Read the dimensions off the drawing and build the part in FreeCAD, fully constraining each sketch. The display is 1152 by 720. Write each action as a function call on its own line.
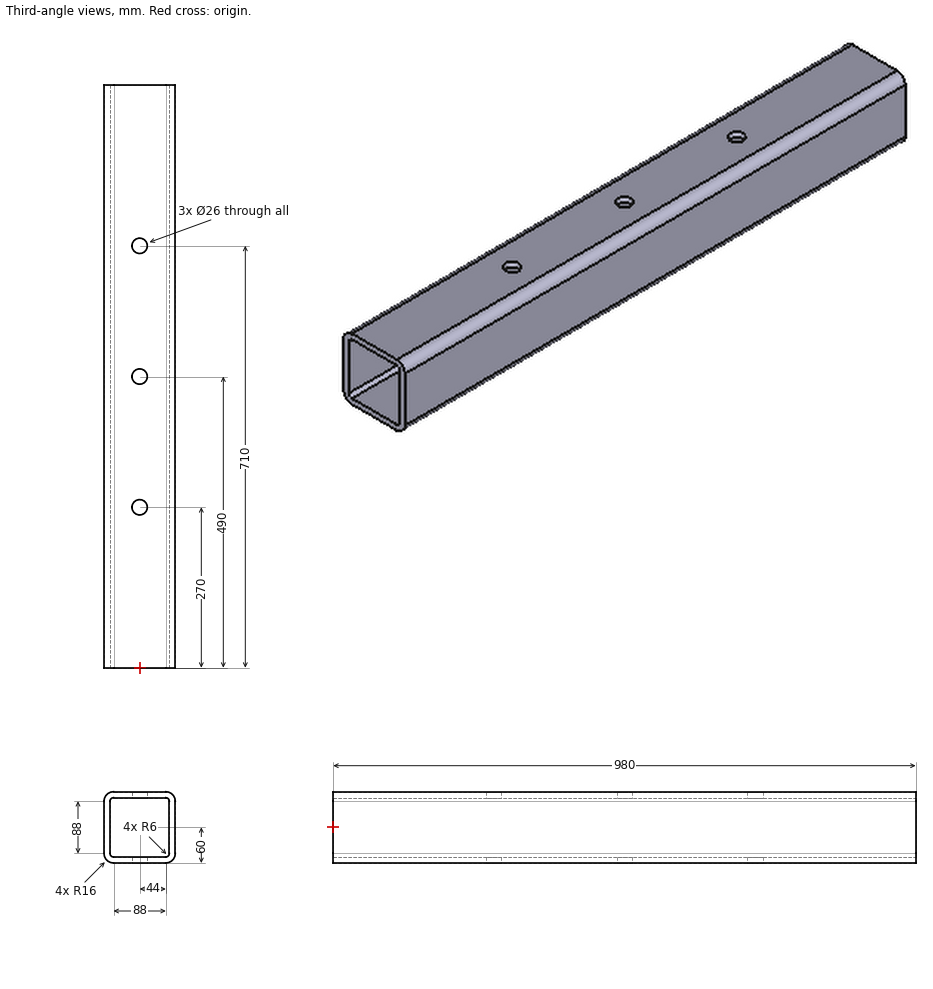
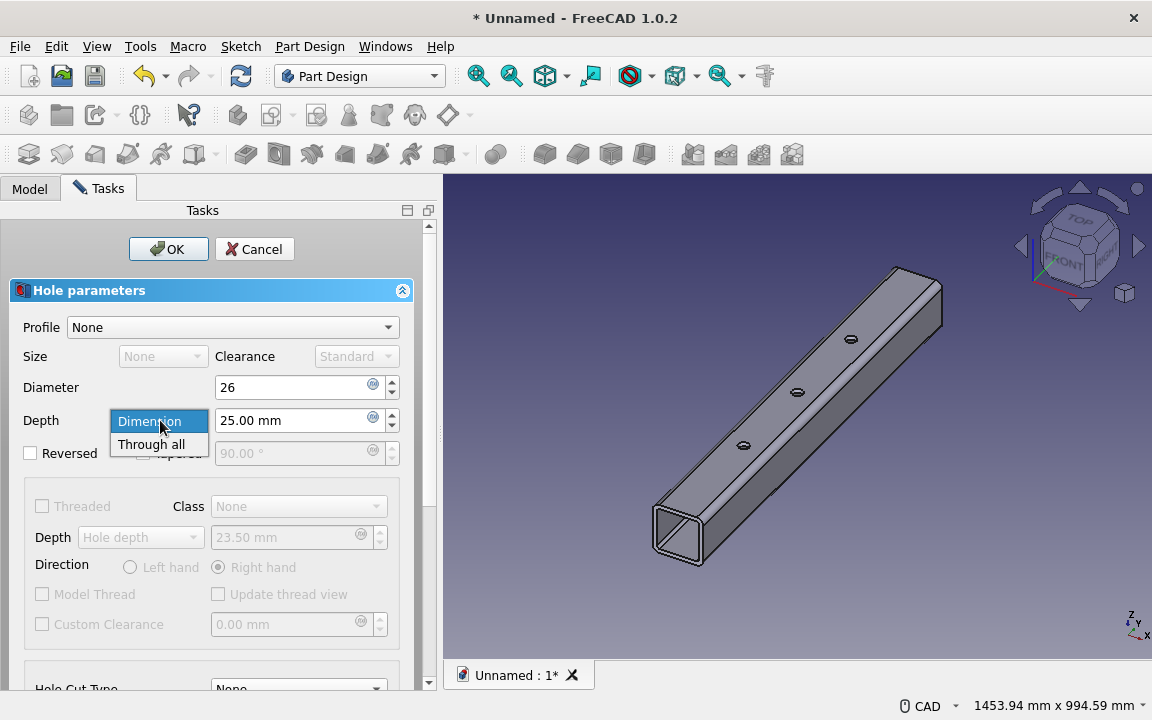
click(158, 444)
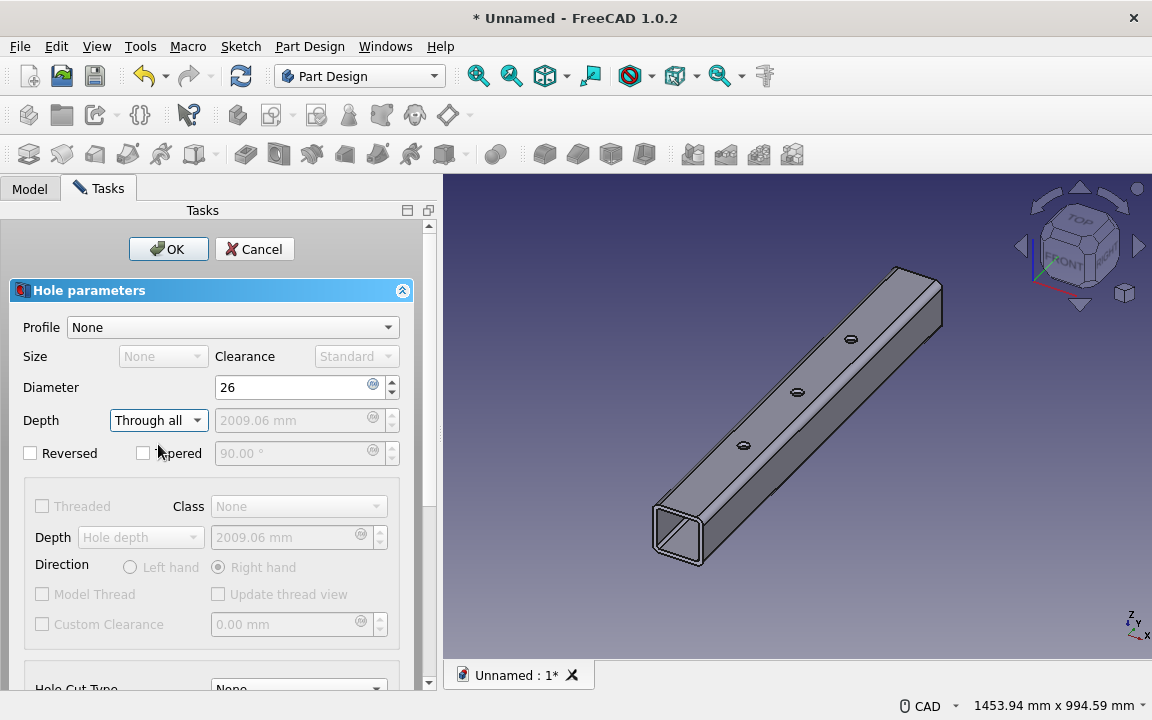
click(169, 249)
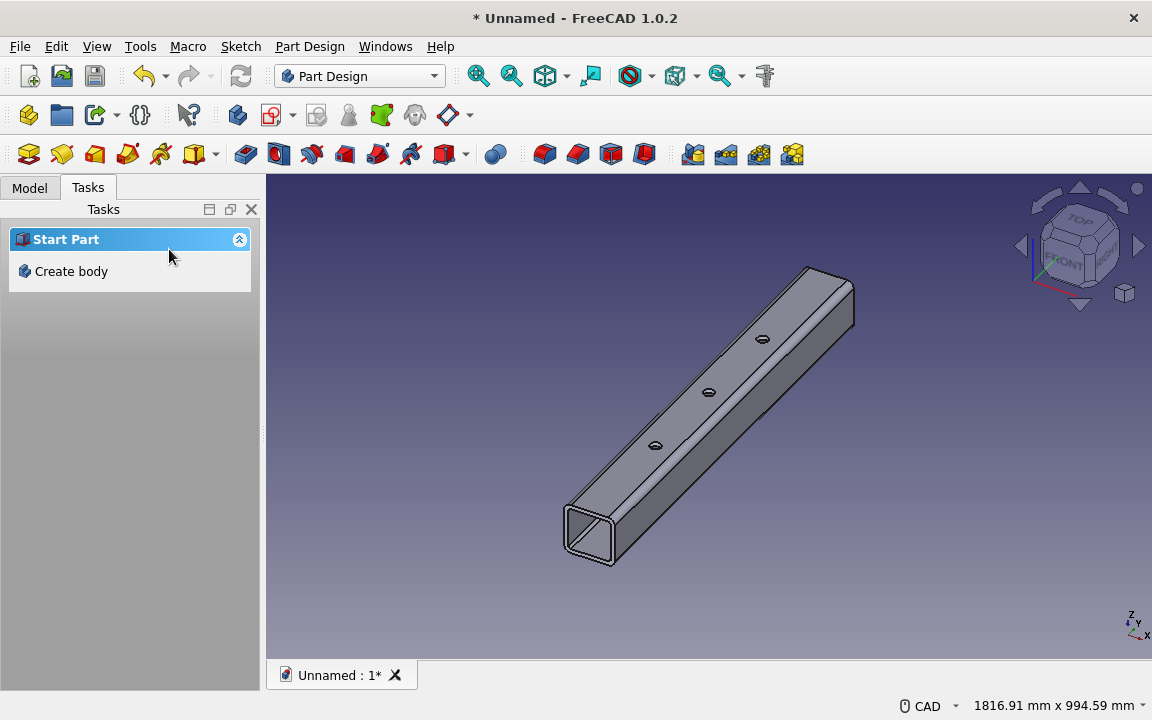
key(0)